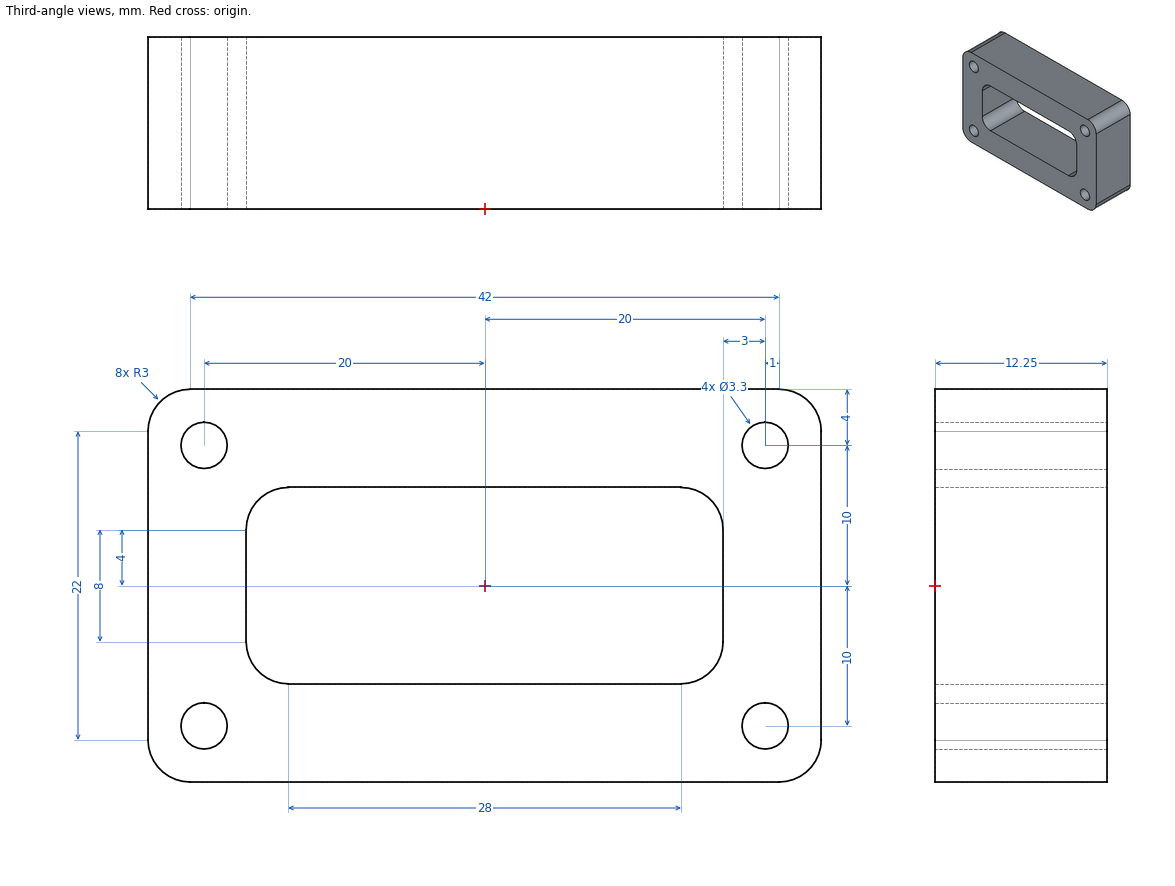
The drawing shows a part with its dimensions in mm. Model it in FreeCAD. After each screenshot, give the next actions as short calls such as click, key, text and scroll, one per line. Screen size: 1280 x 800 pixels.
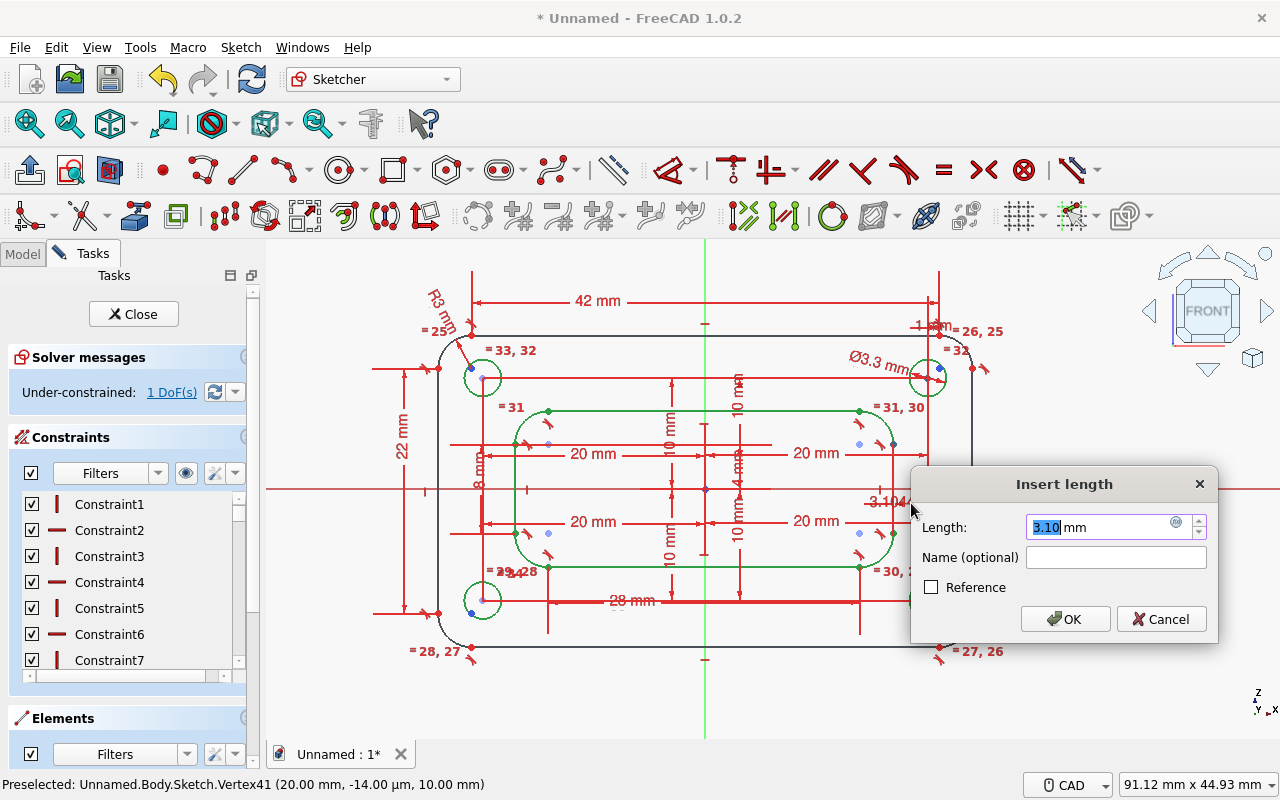
text(3)
key(Return)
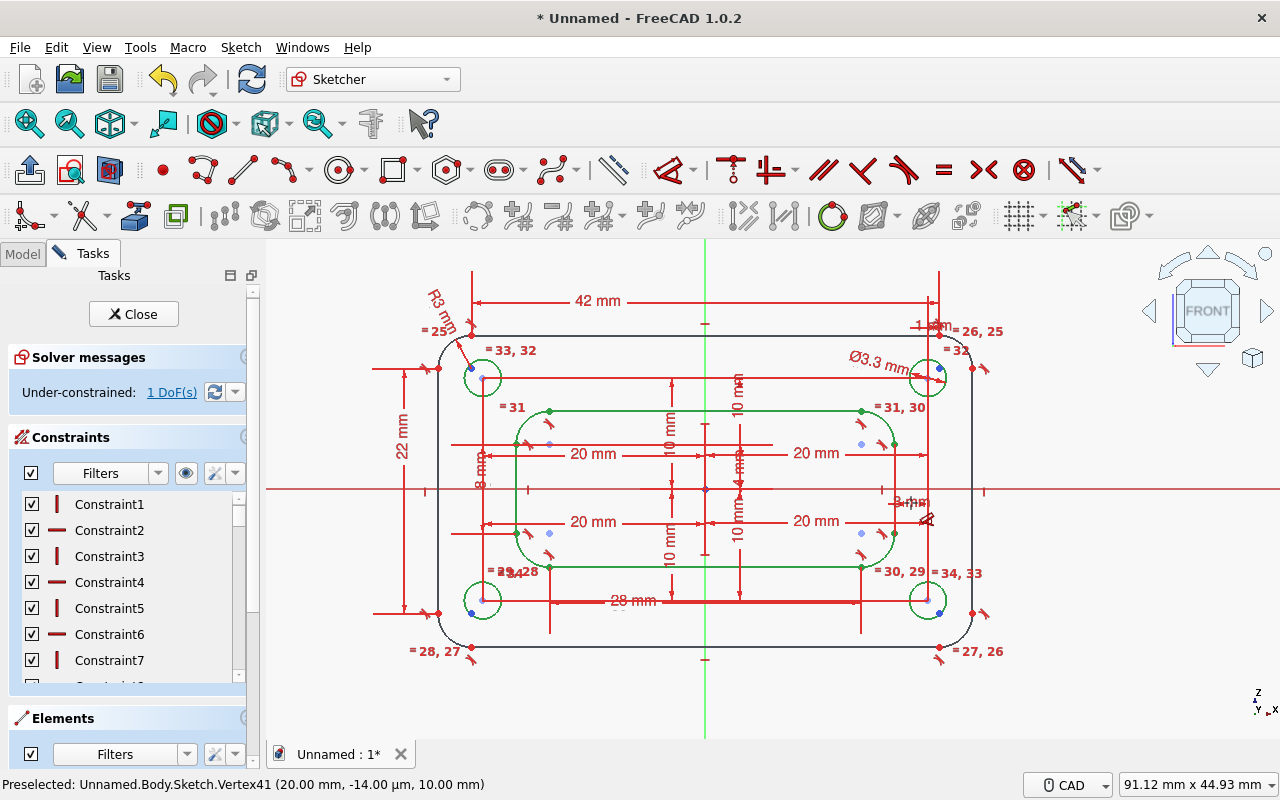
click(939, 336)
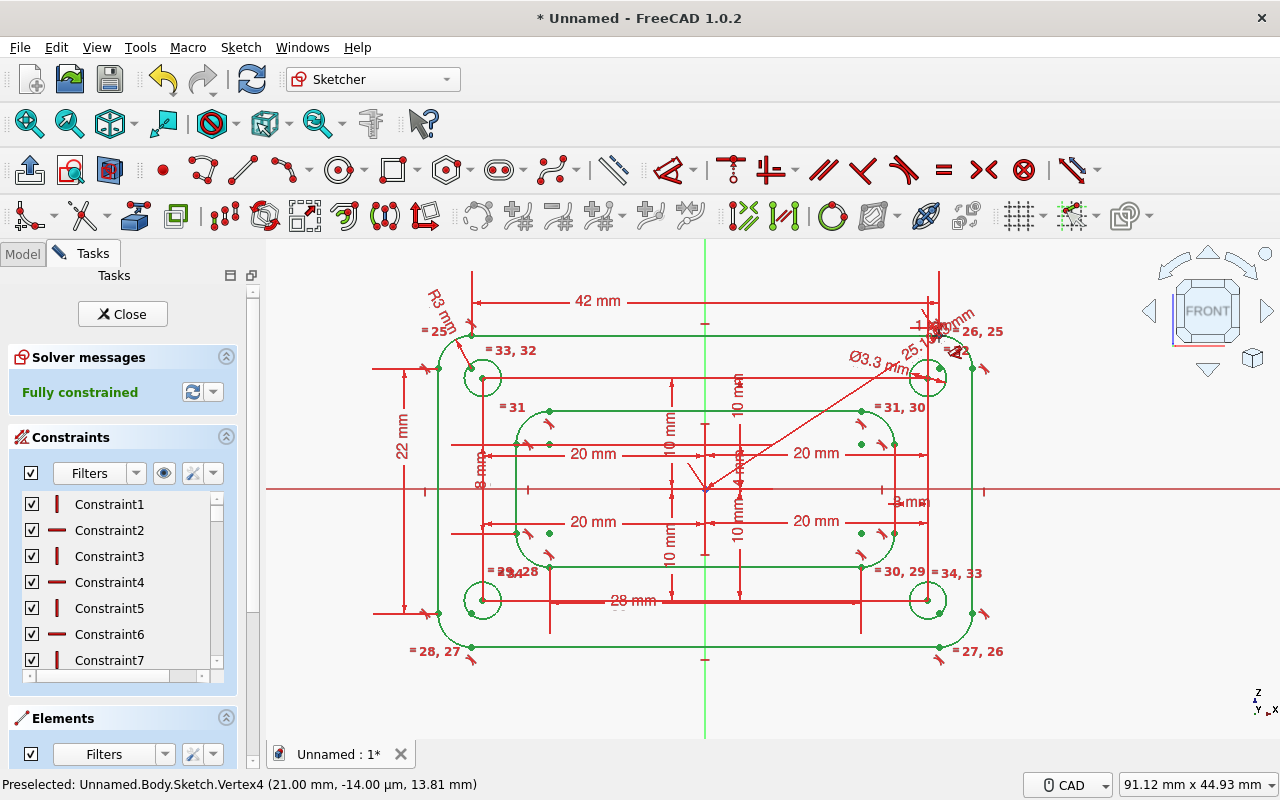
click(928, 378)
click(997, 357)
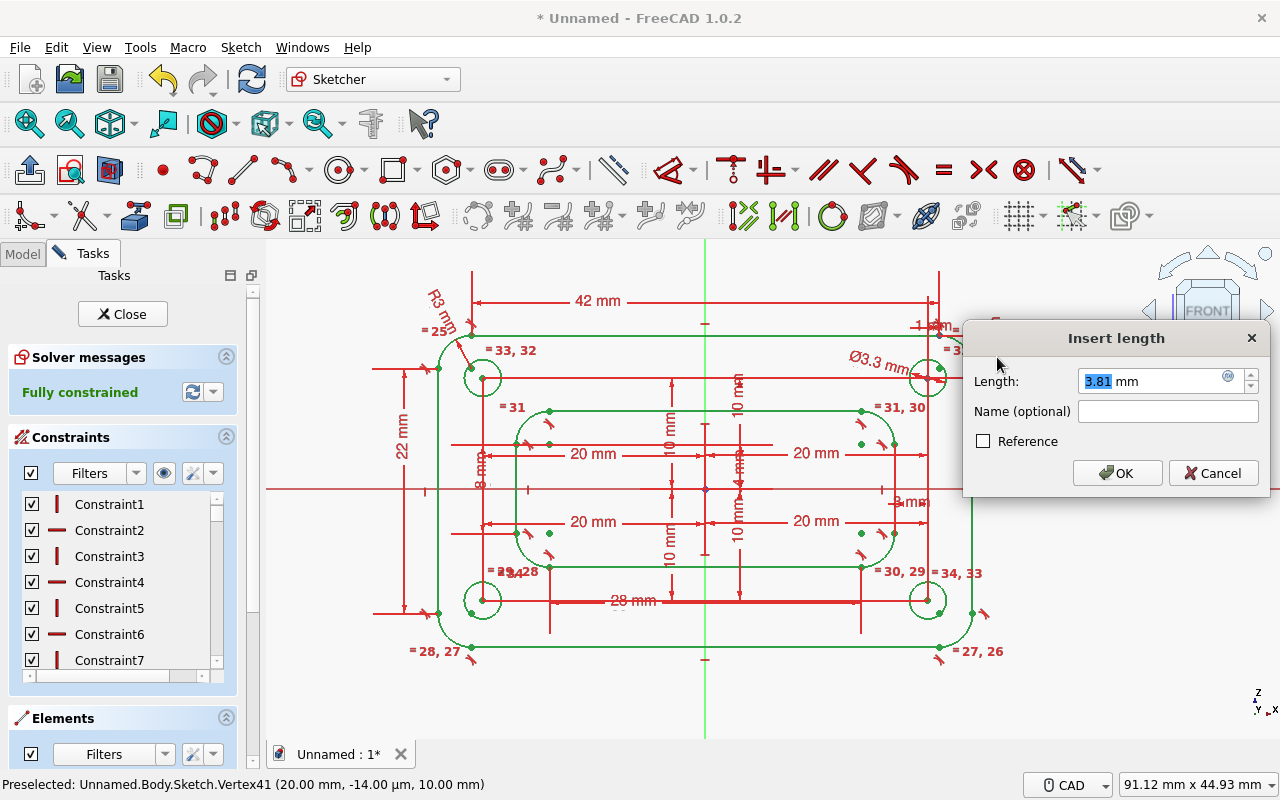
text(4)
key(Return)
key(Escape)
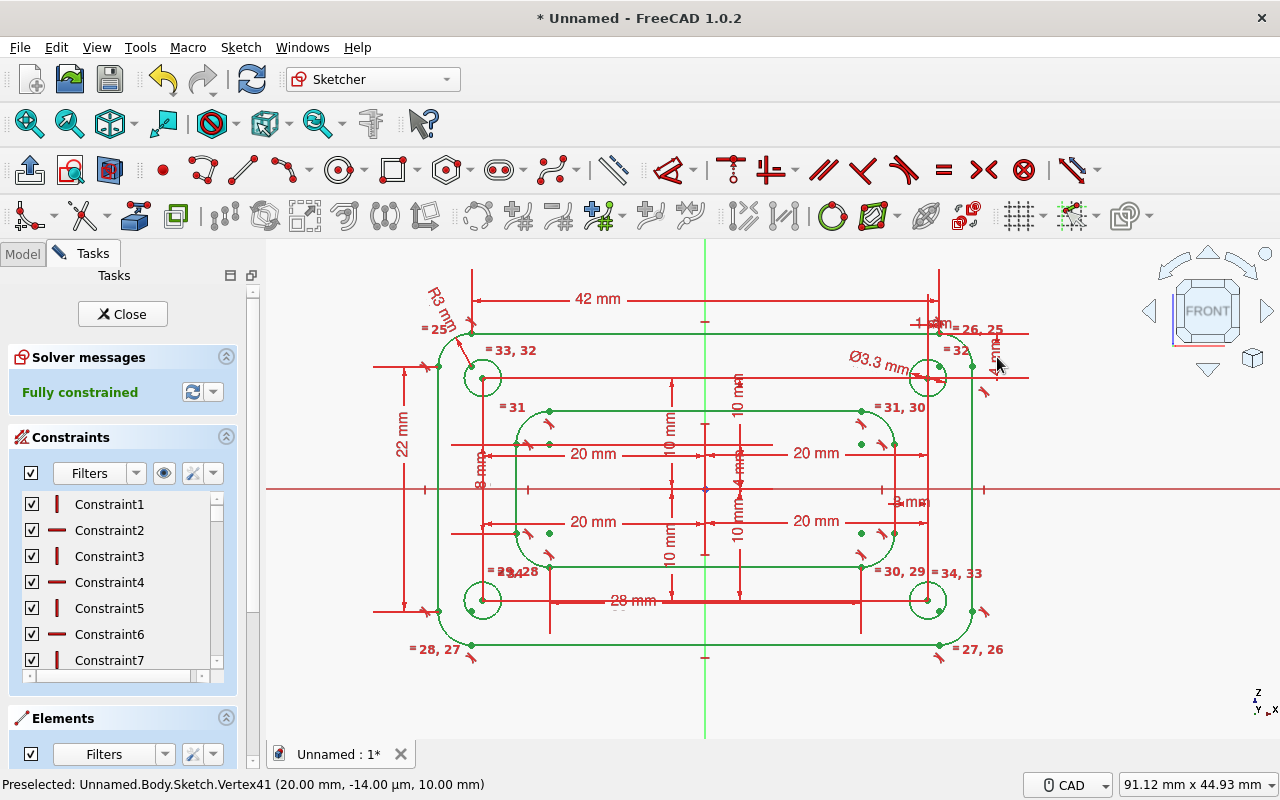
click(123, 314)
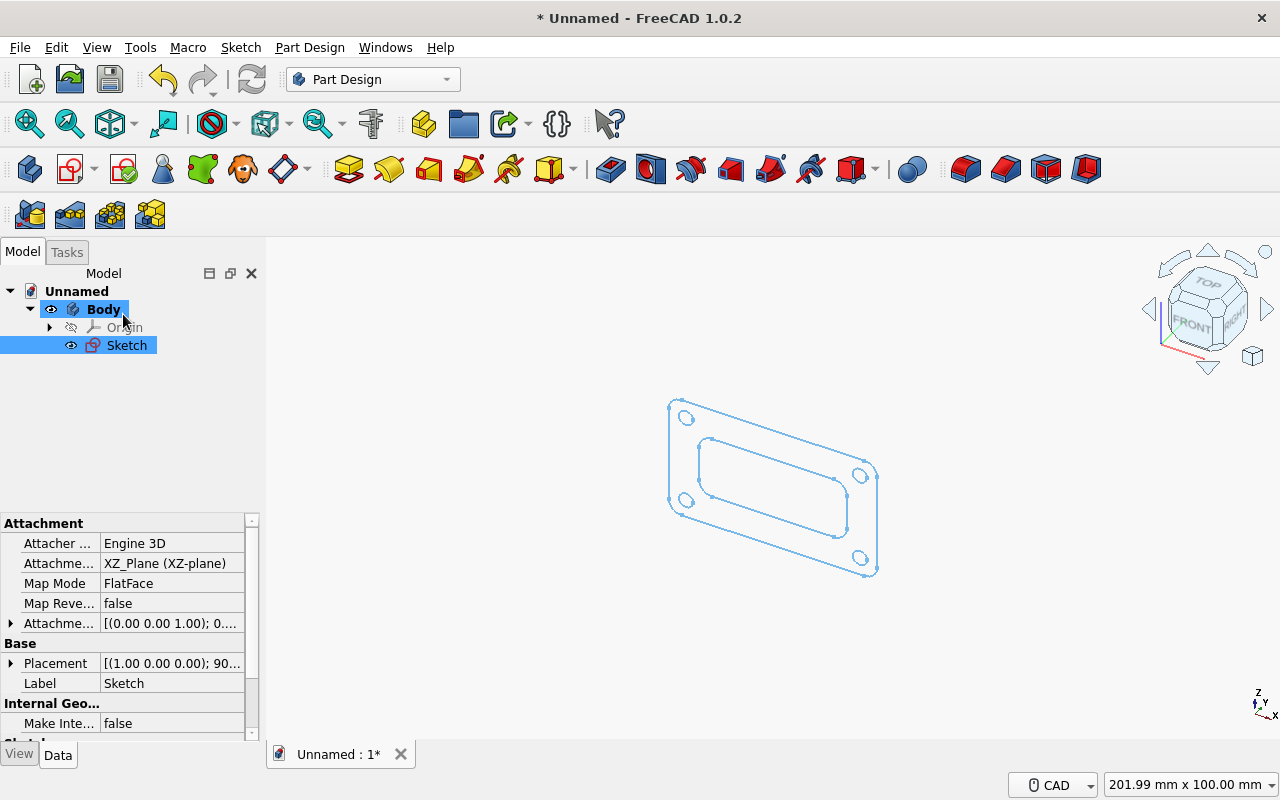
click(350, 170)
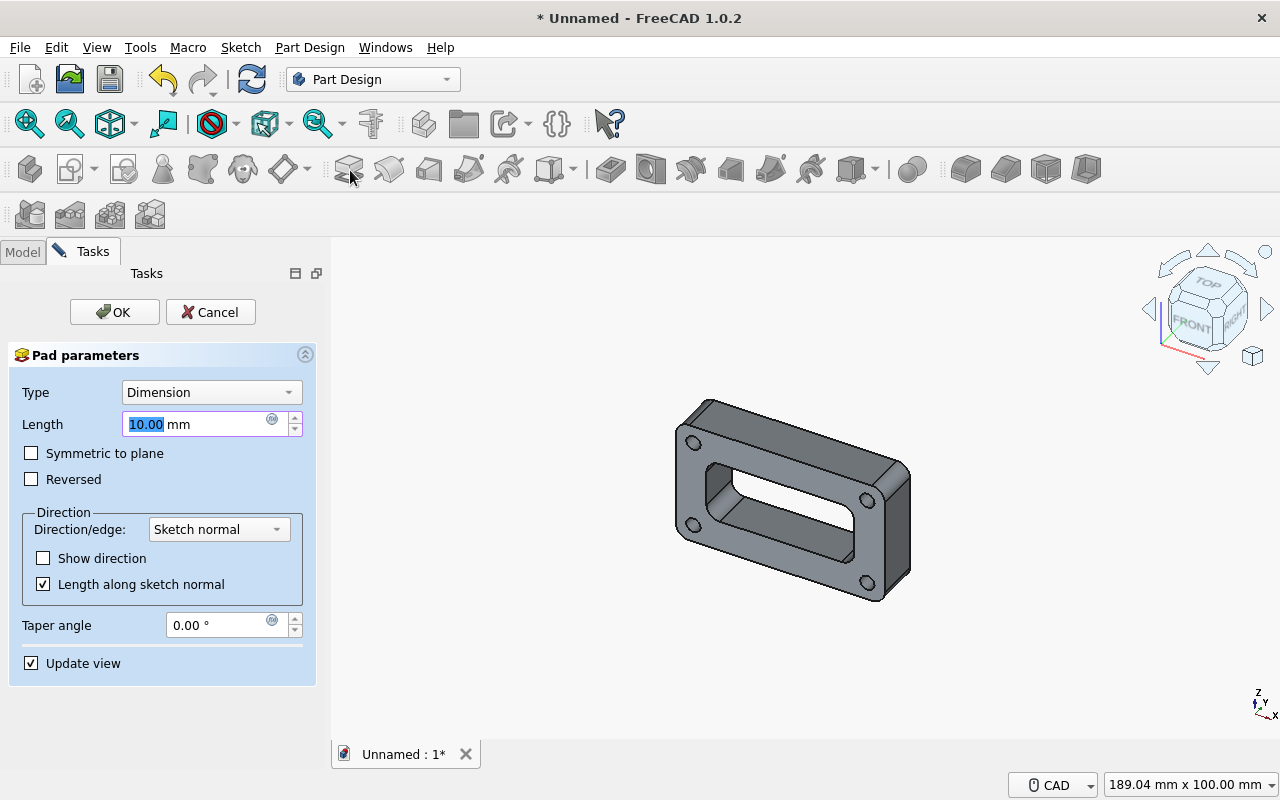
text(12.25)
key(Tab)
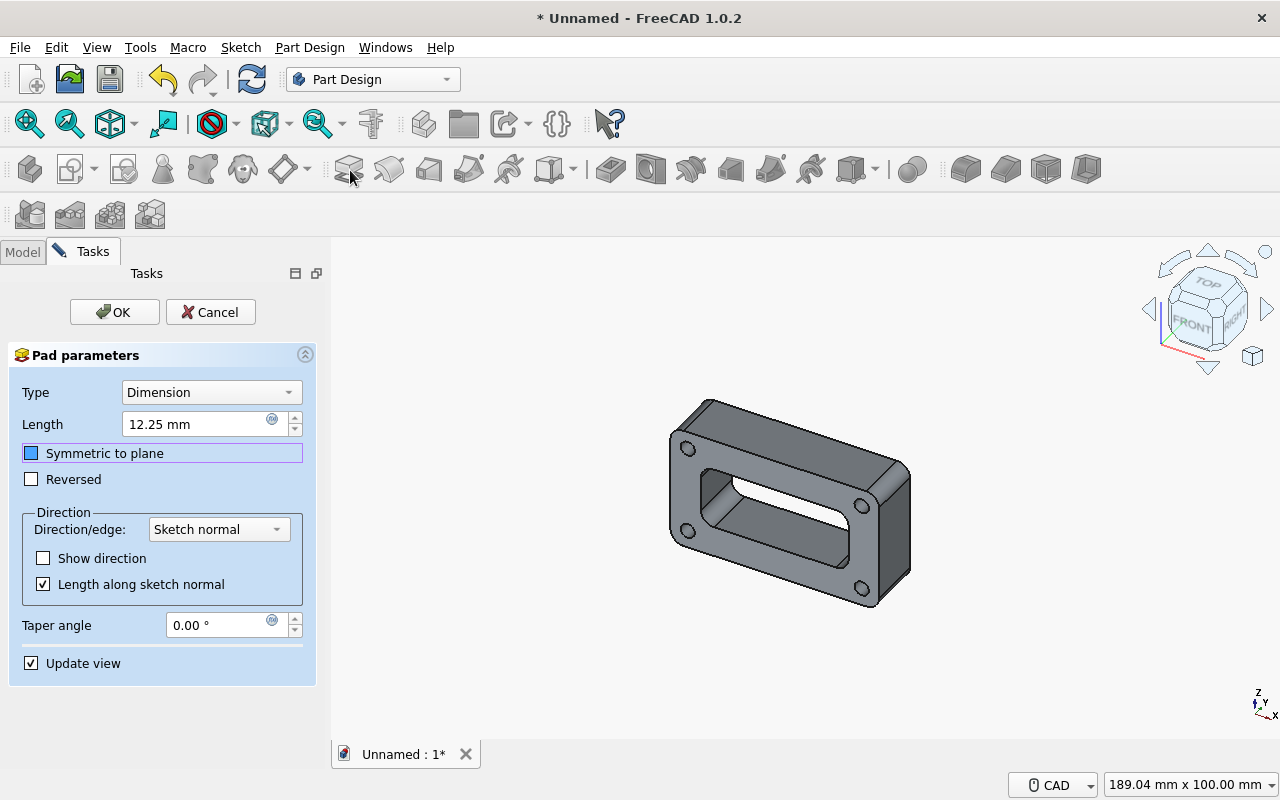
click(30, 479)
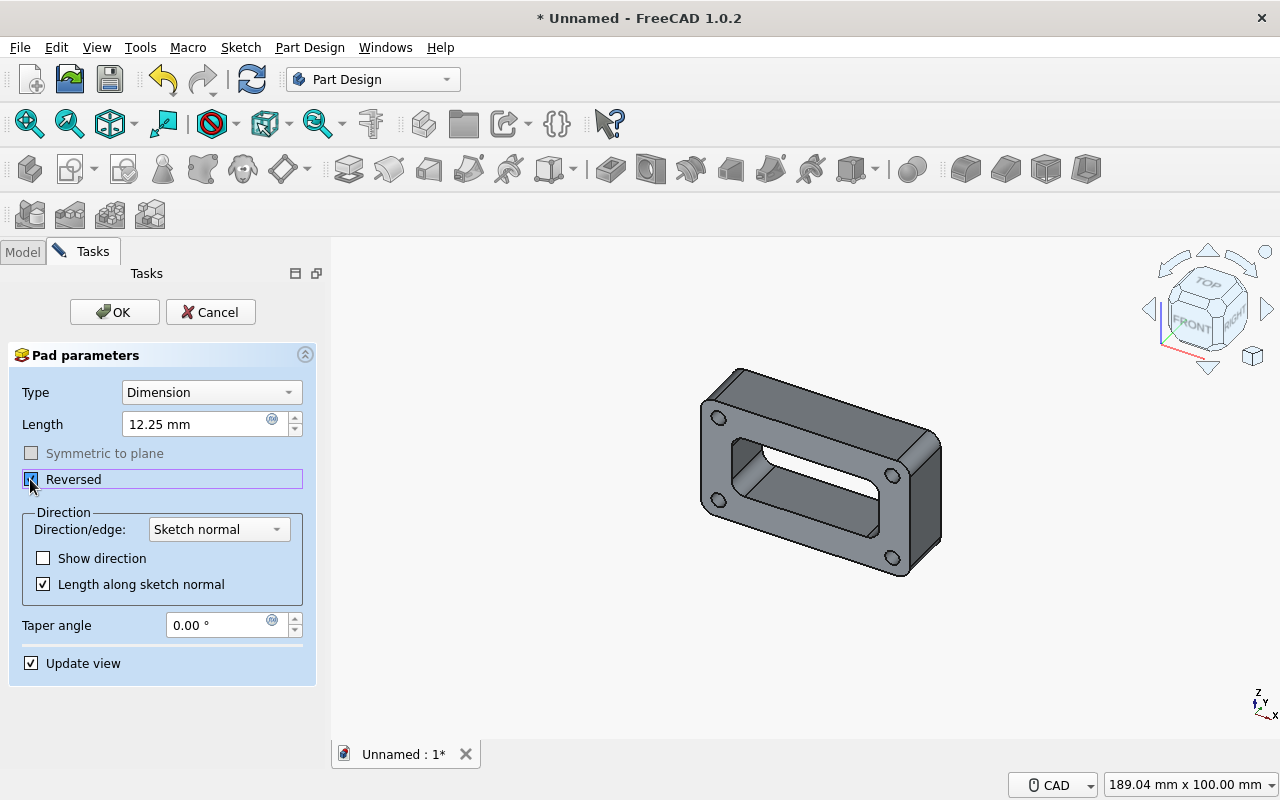
click(115, 312)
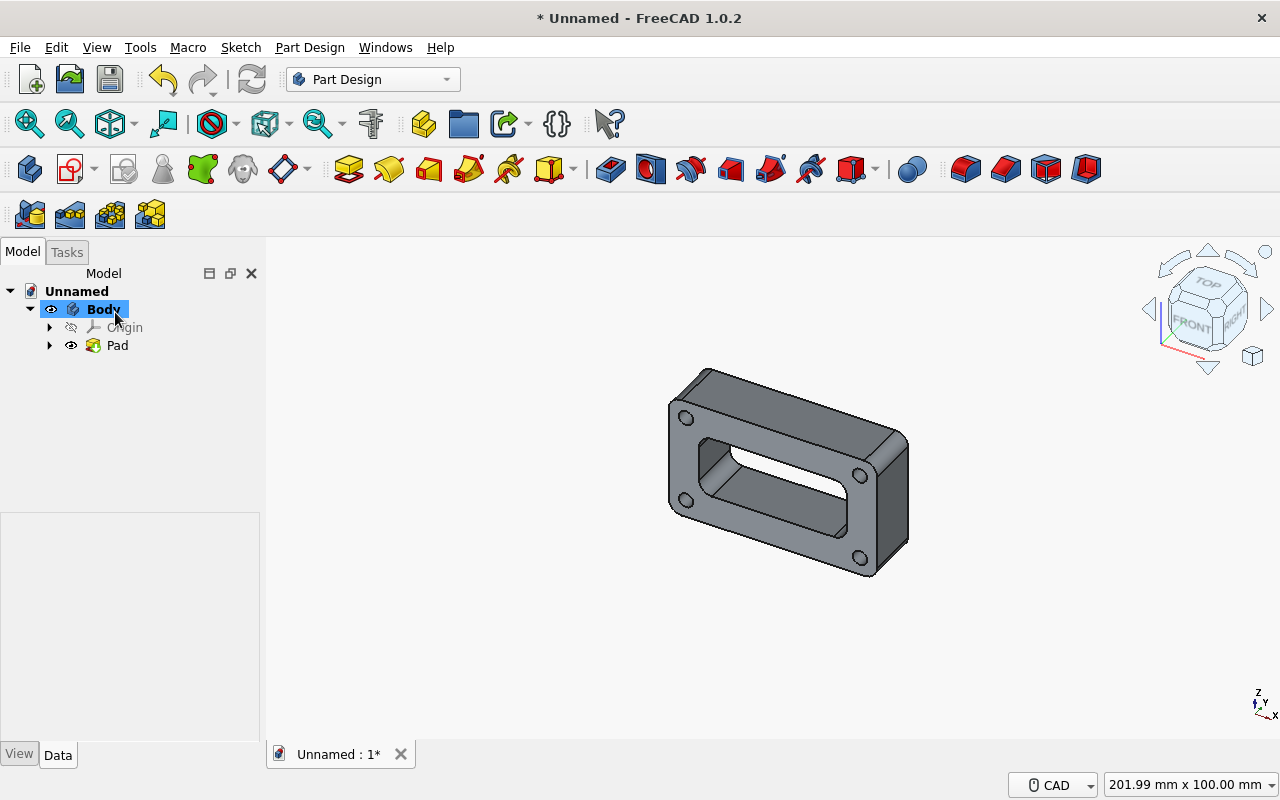
key(0)